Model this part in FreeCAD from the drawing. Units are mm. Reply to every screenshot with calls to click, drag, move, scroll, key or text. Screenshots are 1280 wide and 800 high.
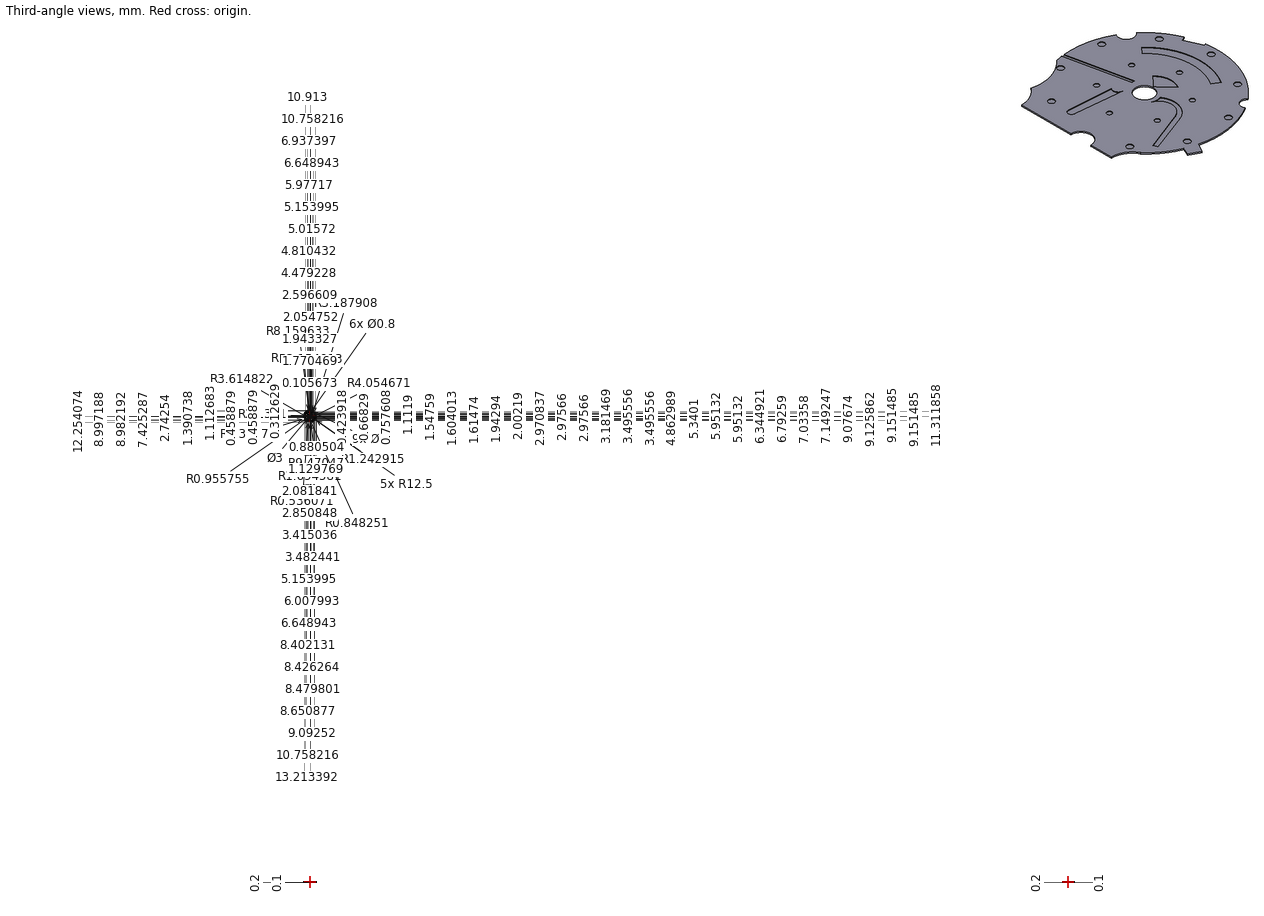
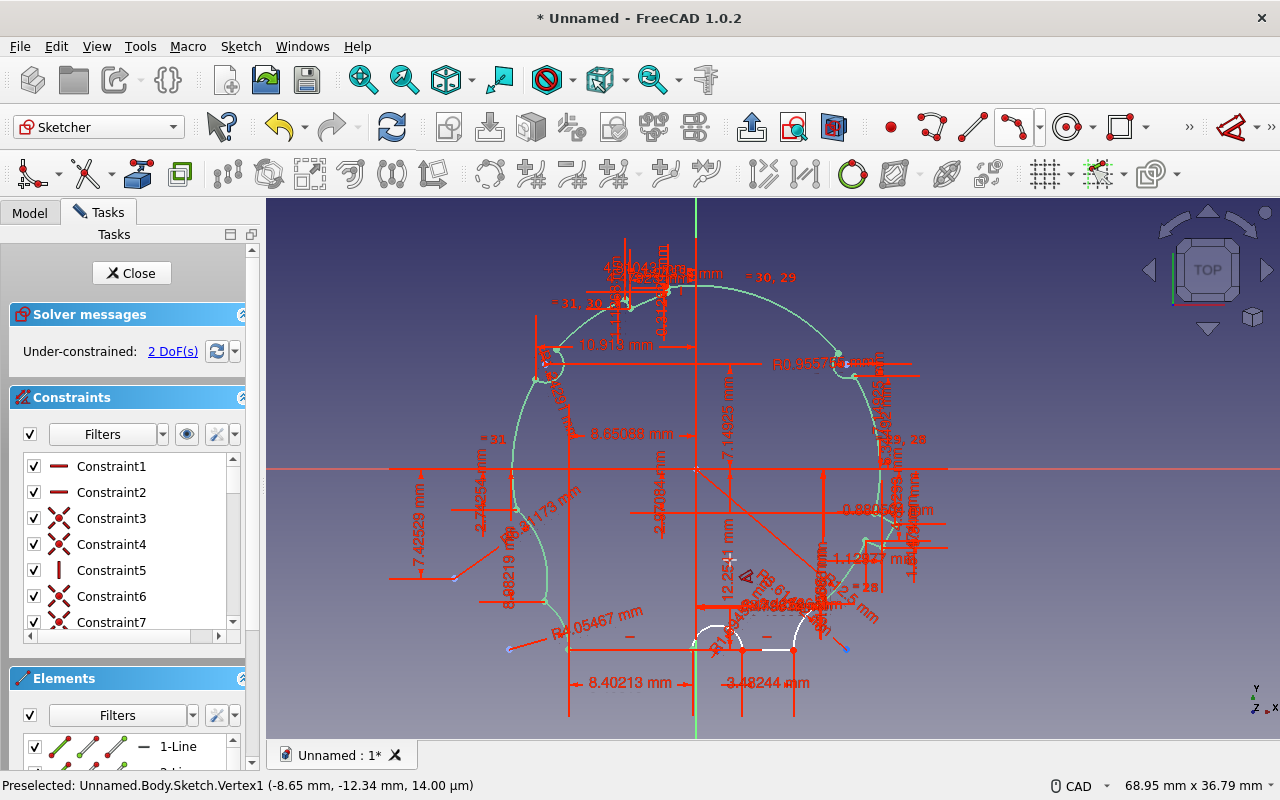
click(742, 650)
click(776, 518)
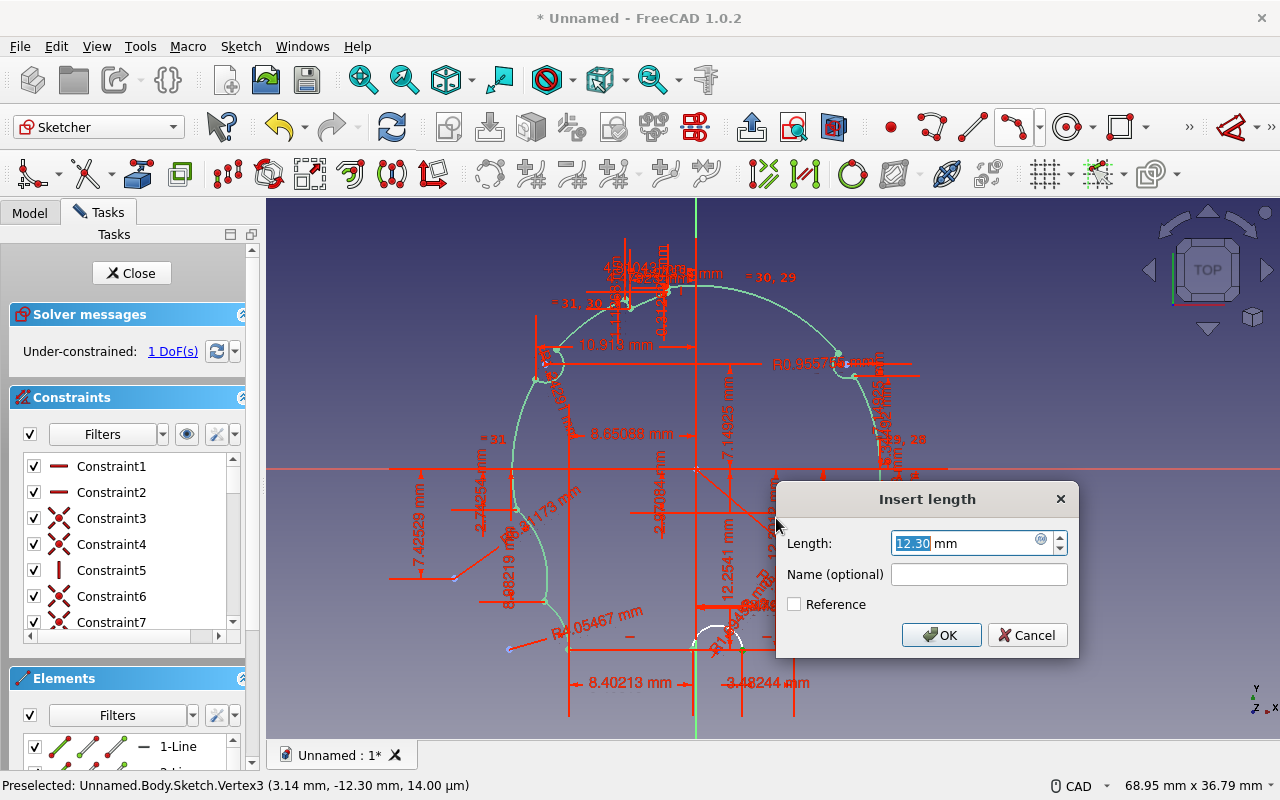
text(12.254074)
key(Return)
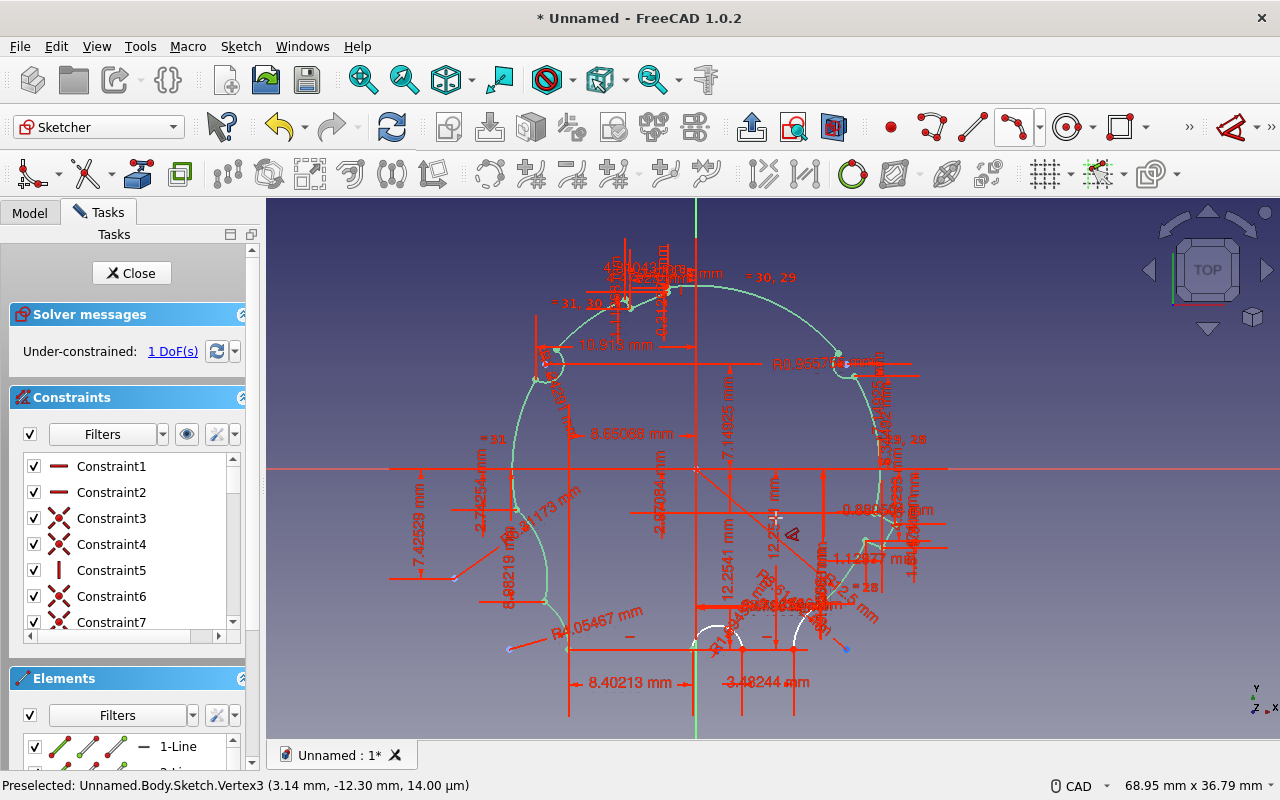
click(717, 650)
click(751, 497)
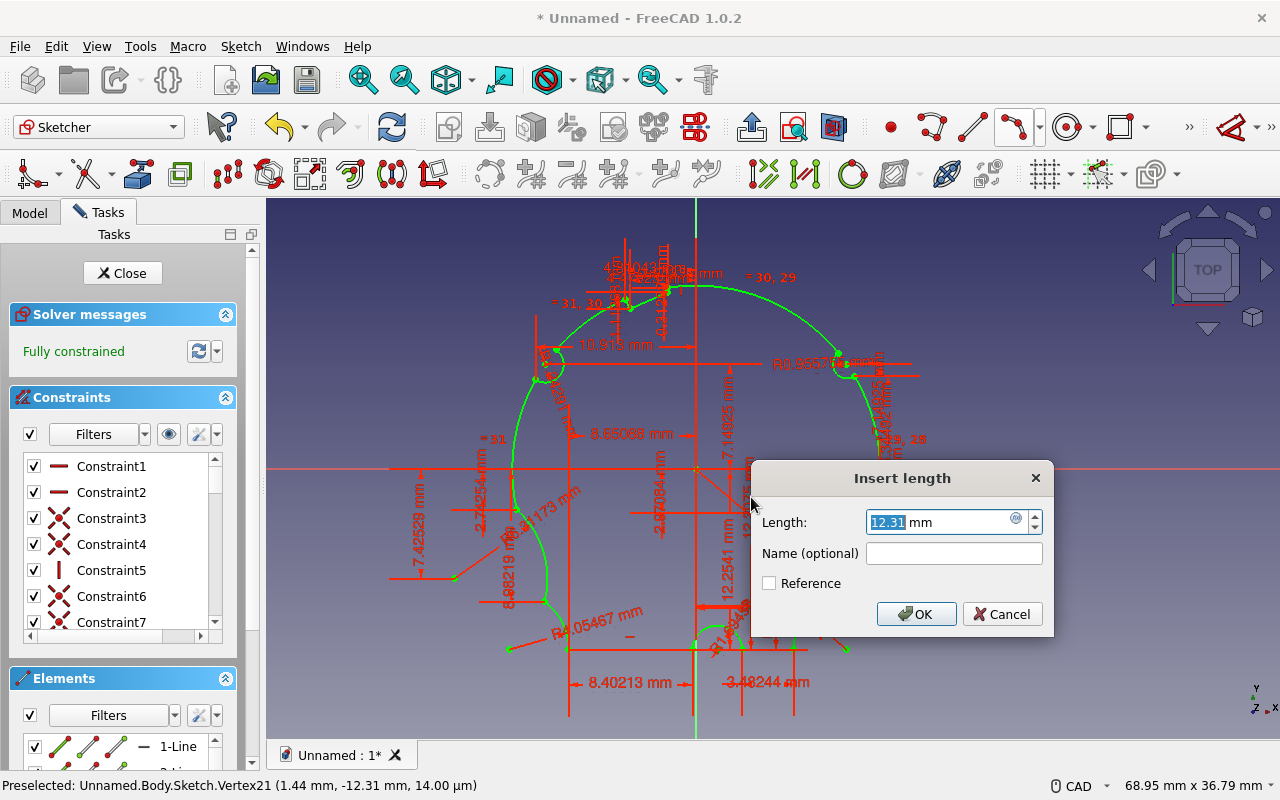
text(12.254074)
key(Return)
key(Escape)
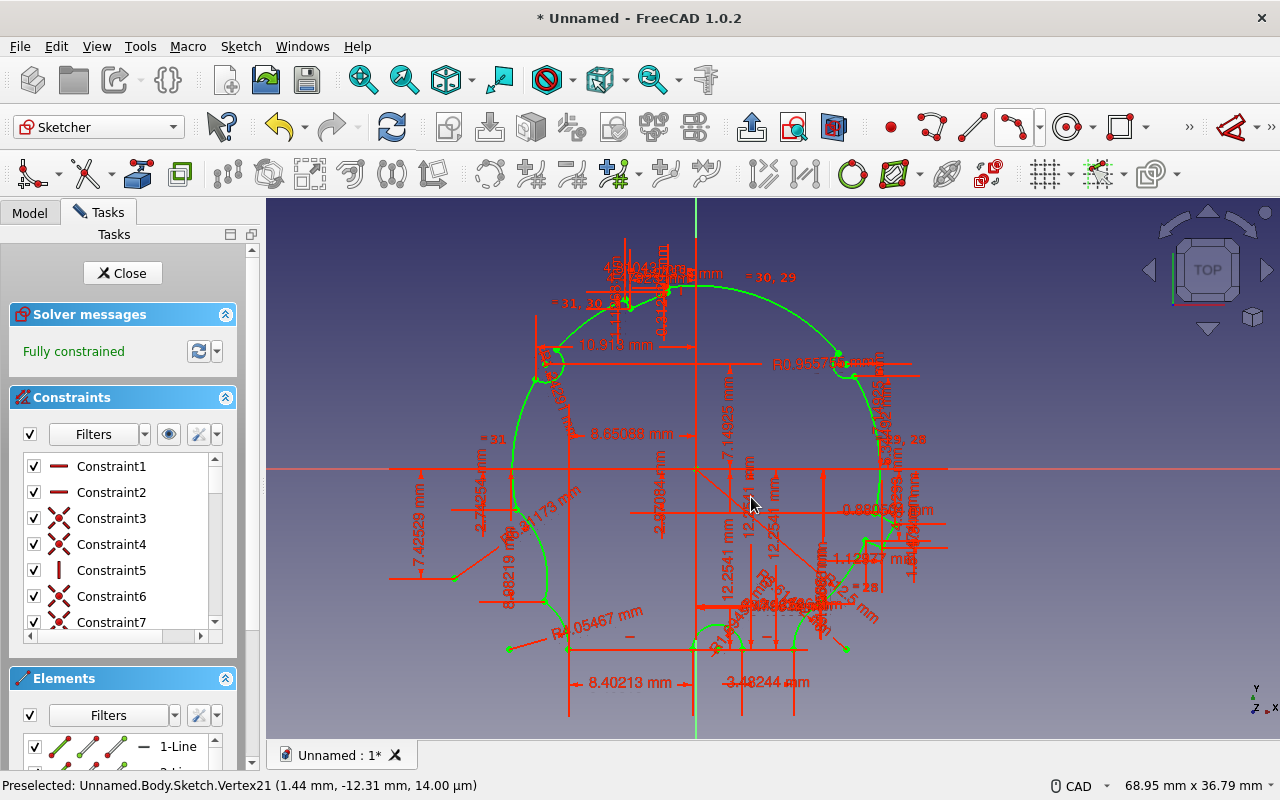
click(123, 273)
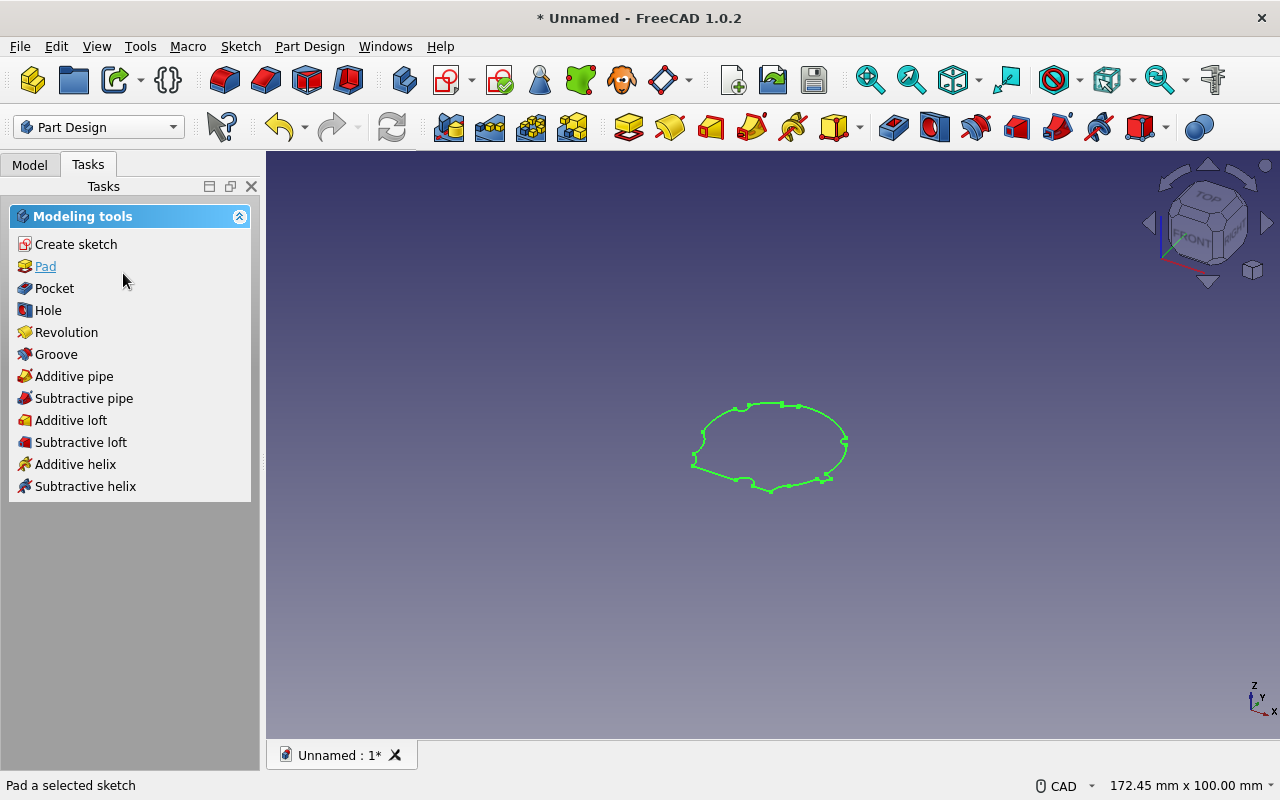
click(629, 128)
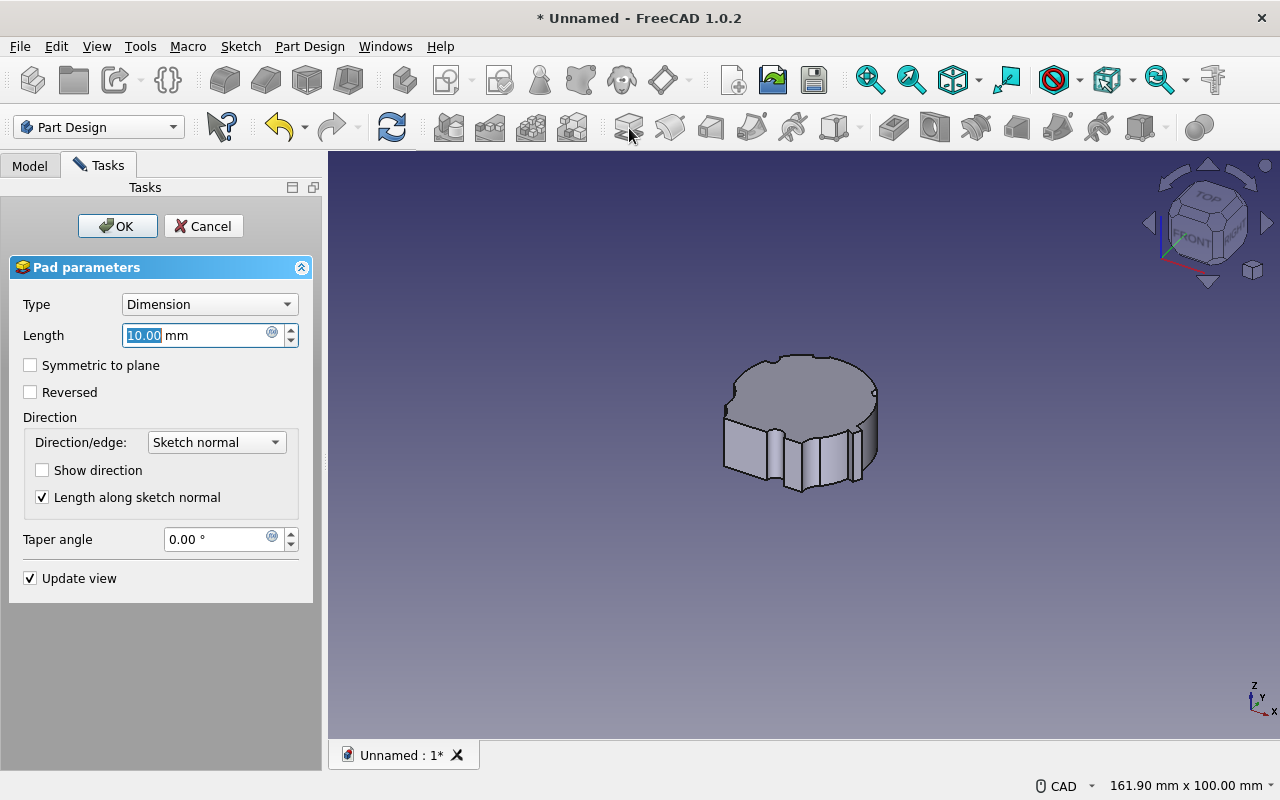
text(0.2)
key(Tab)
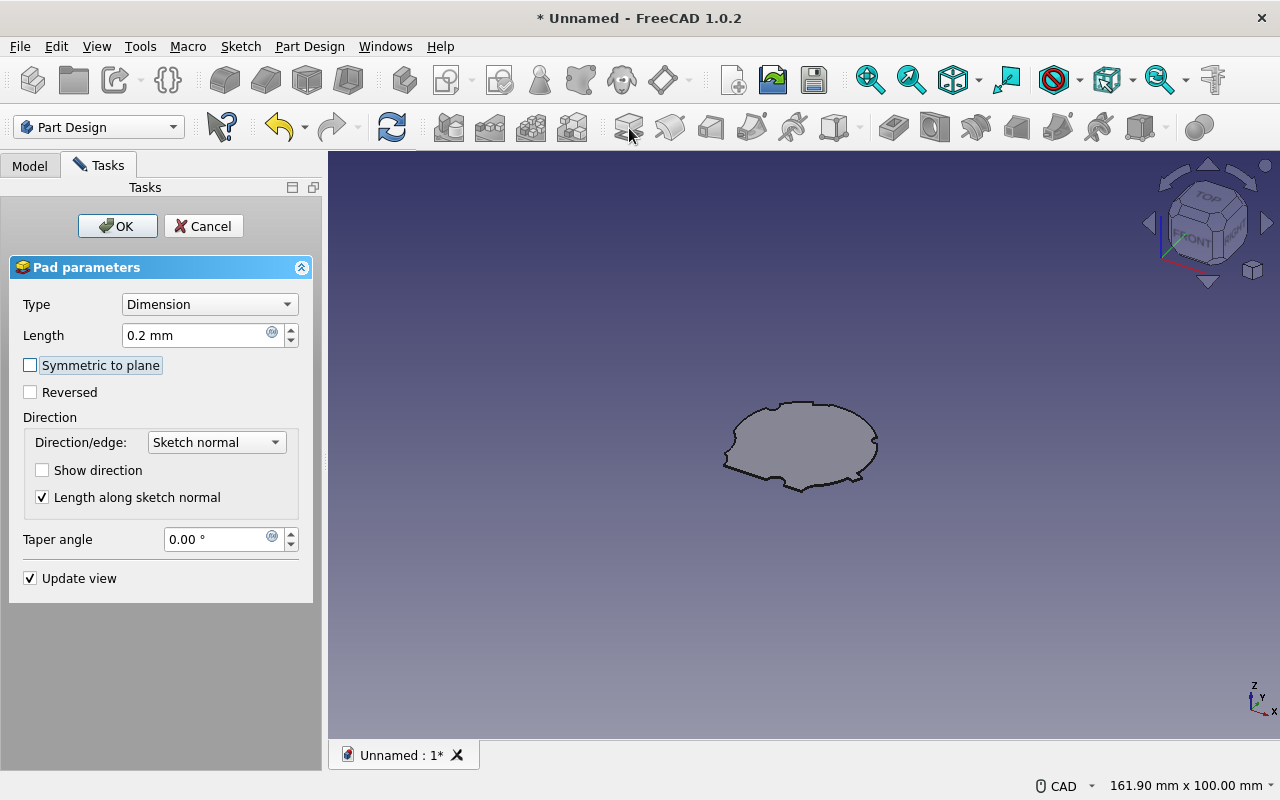
click(118, 226)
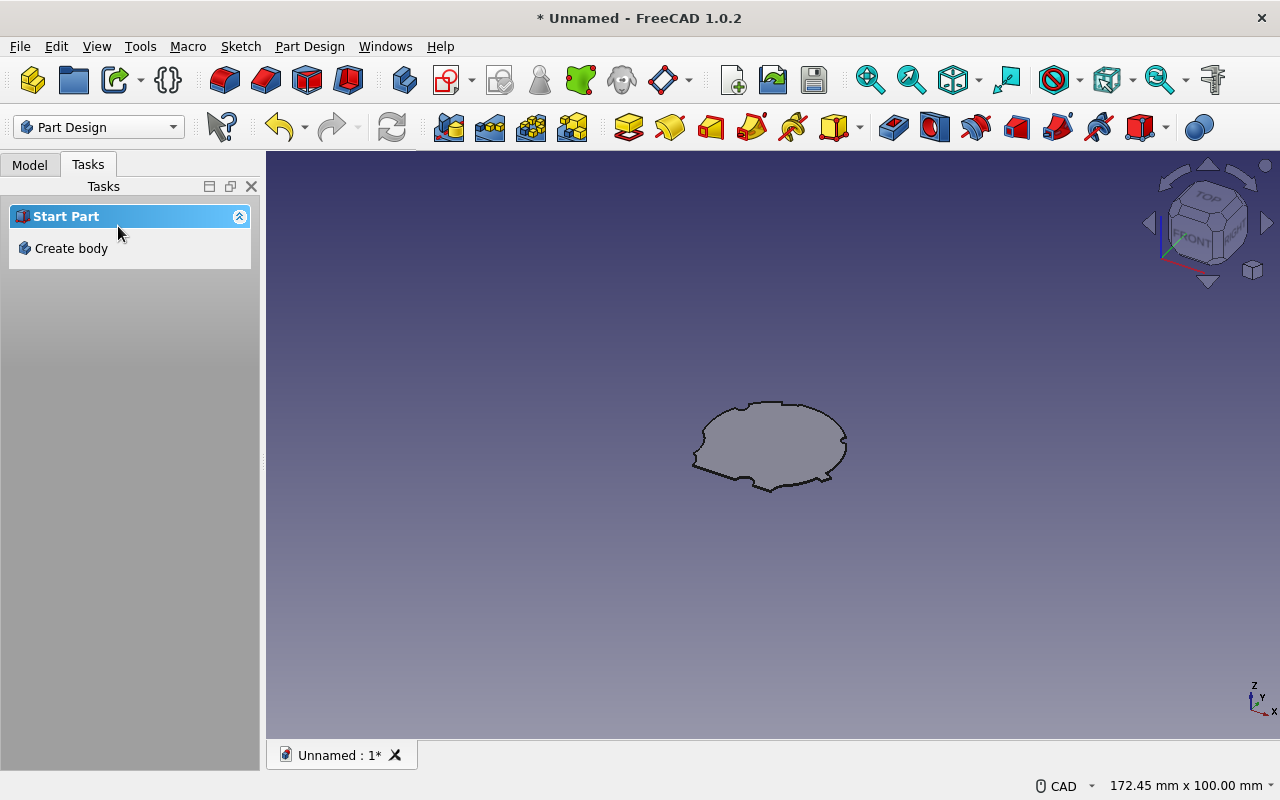
key(v)
key(f)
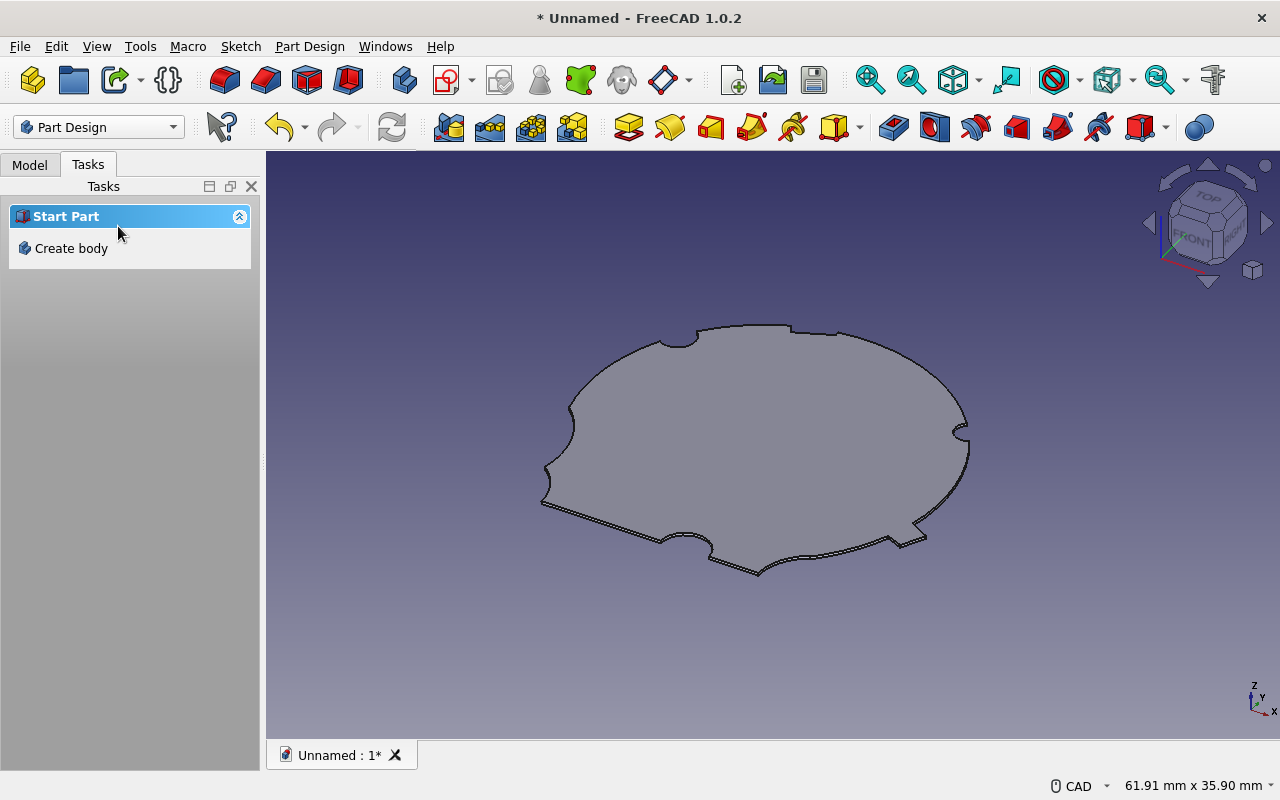
click(773, 443)